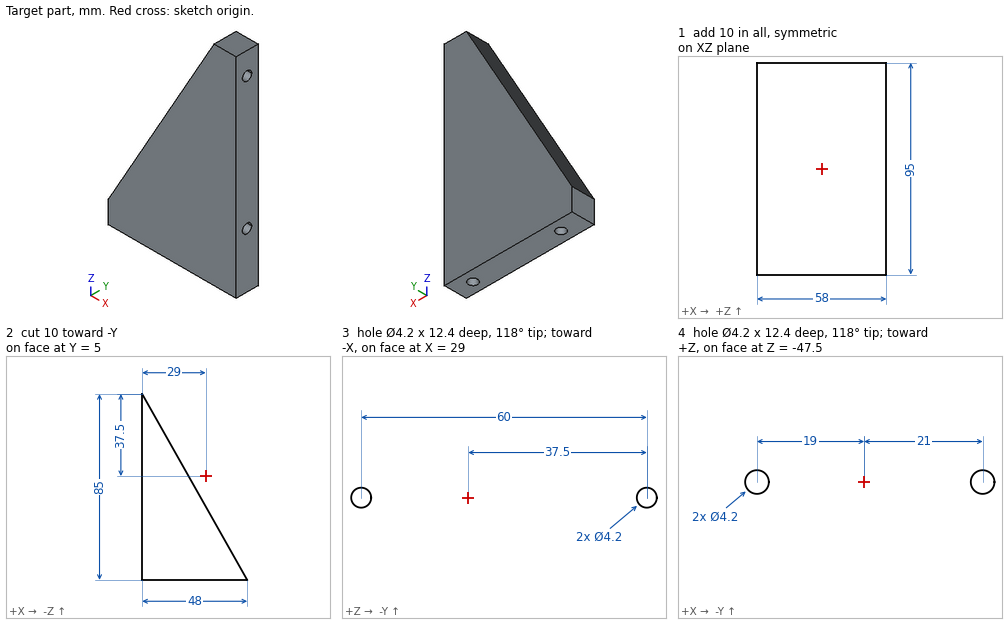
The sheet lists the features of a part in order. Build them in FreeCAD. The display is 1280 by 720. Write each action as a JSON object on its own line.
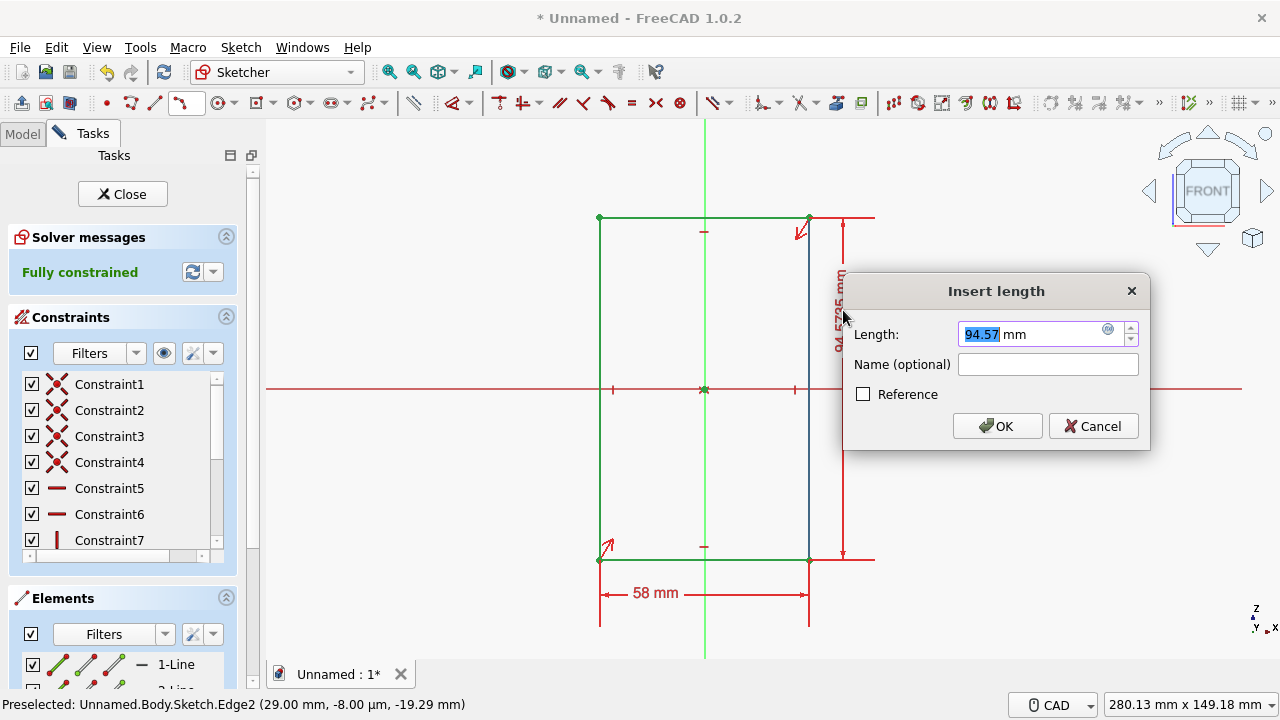
{"action": "type", "text": "95"}
{"action": "key", "text": "Return"}
{"action": "key", "text": "Escape"}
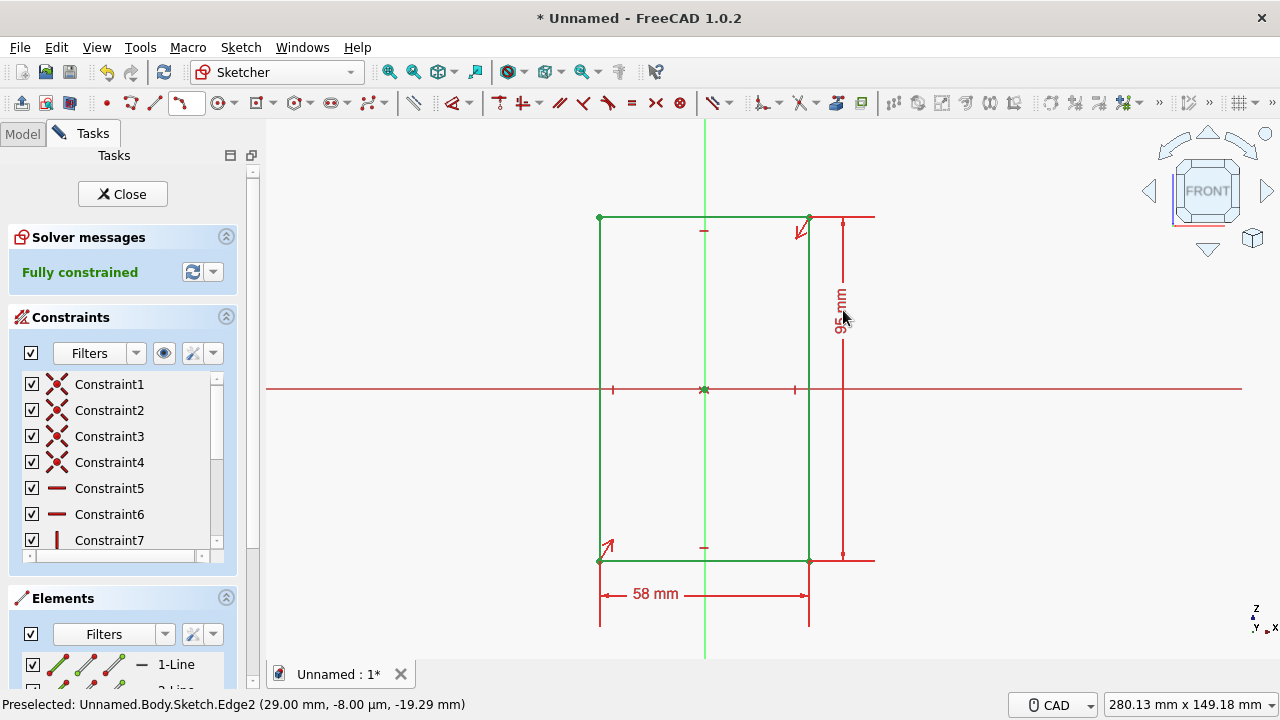
{"action": "left_click", "coordinate": [123, 194]}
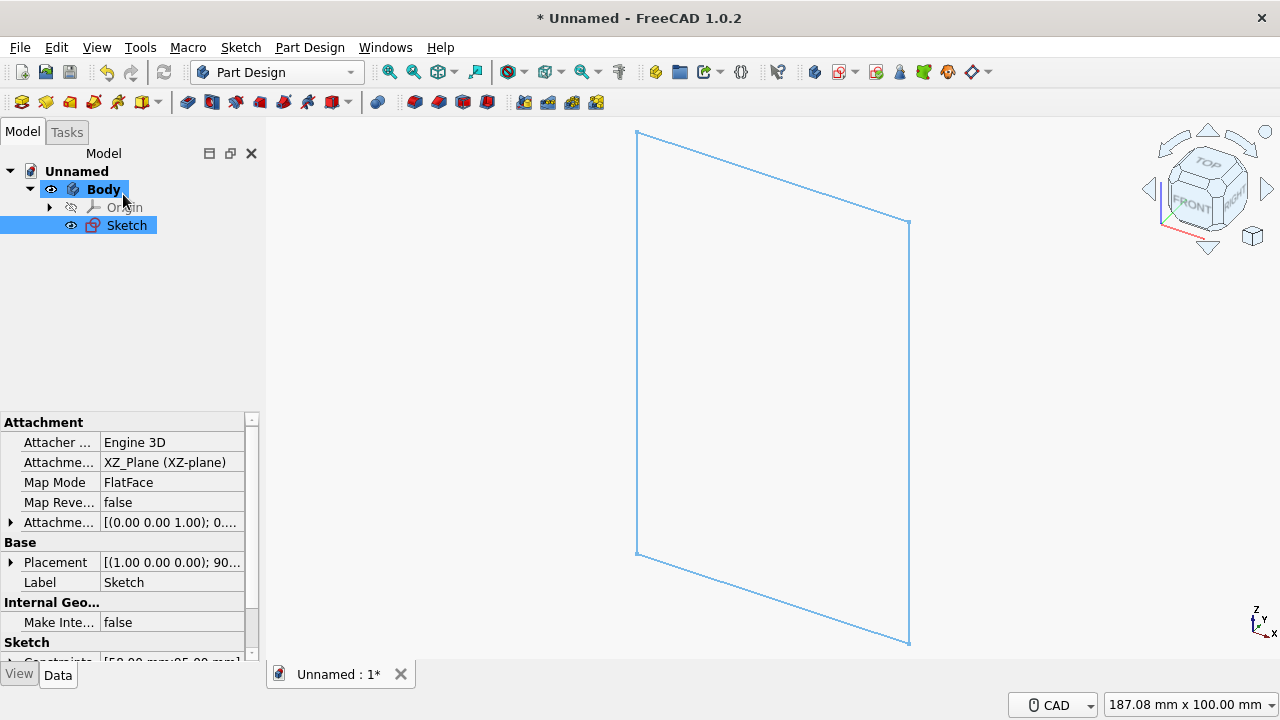
{"action": "left_click", "coordinate": [22, 102]}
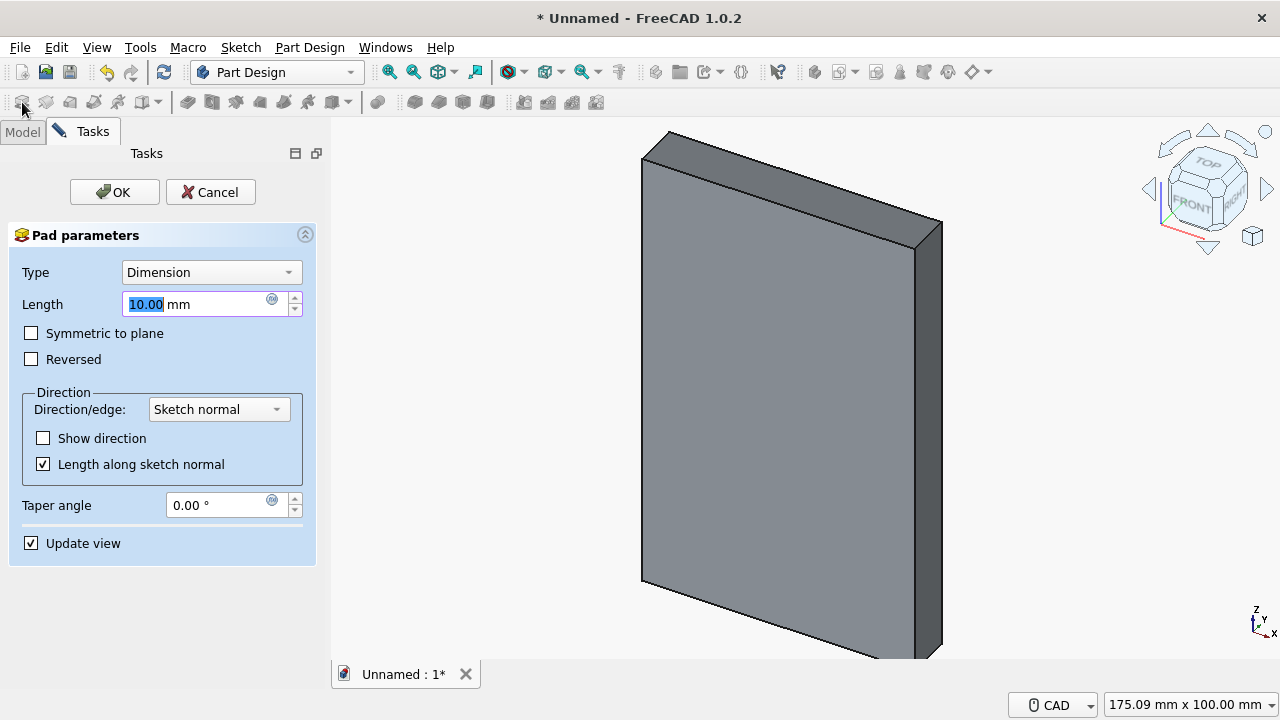
{"action": "type", "text": "10"}
{"action": "key", "text": "Tab"}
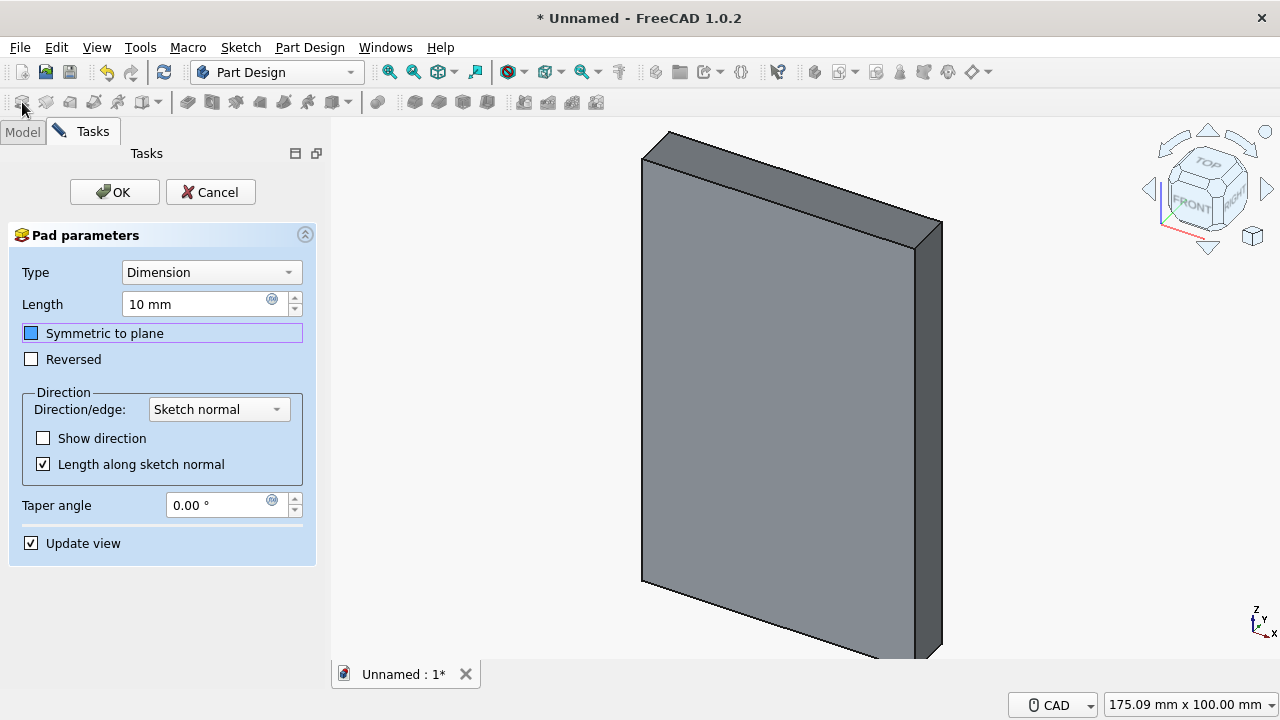
{"action": "left_click", "coordinate": [30, 333]}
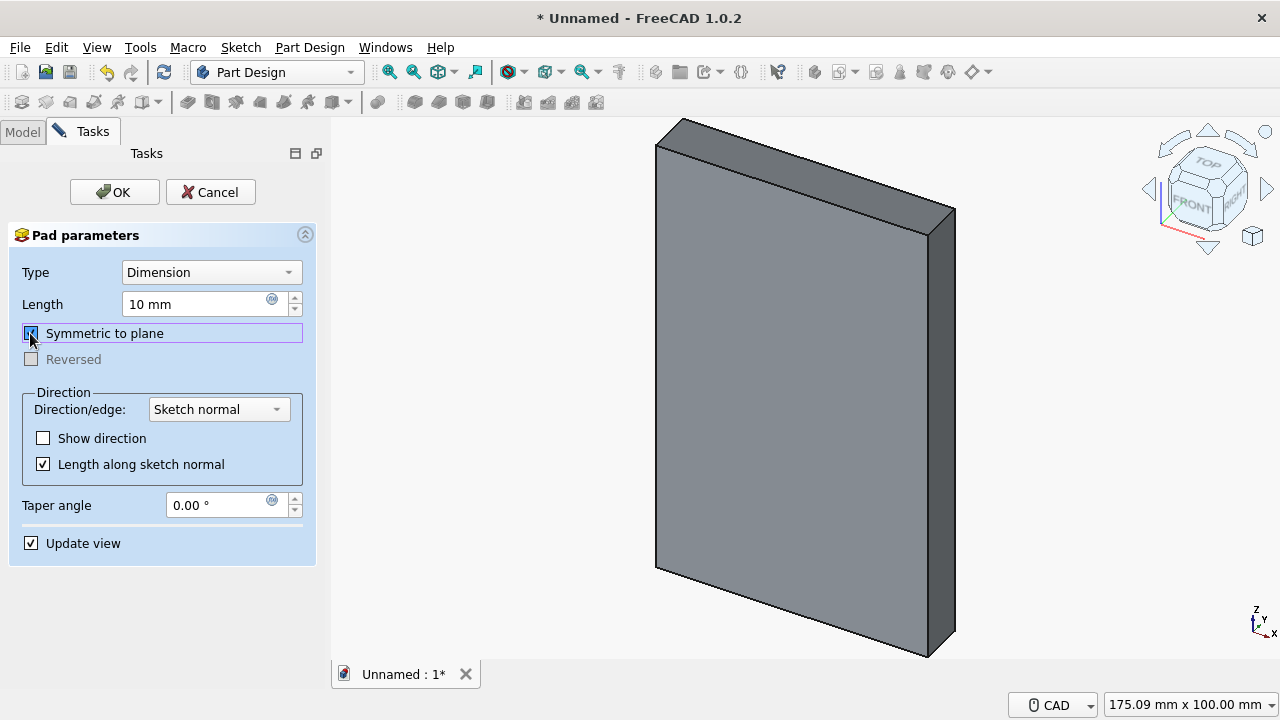
{"action": "left_click", "coordinate": [115, 192]}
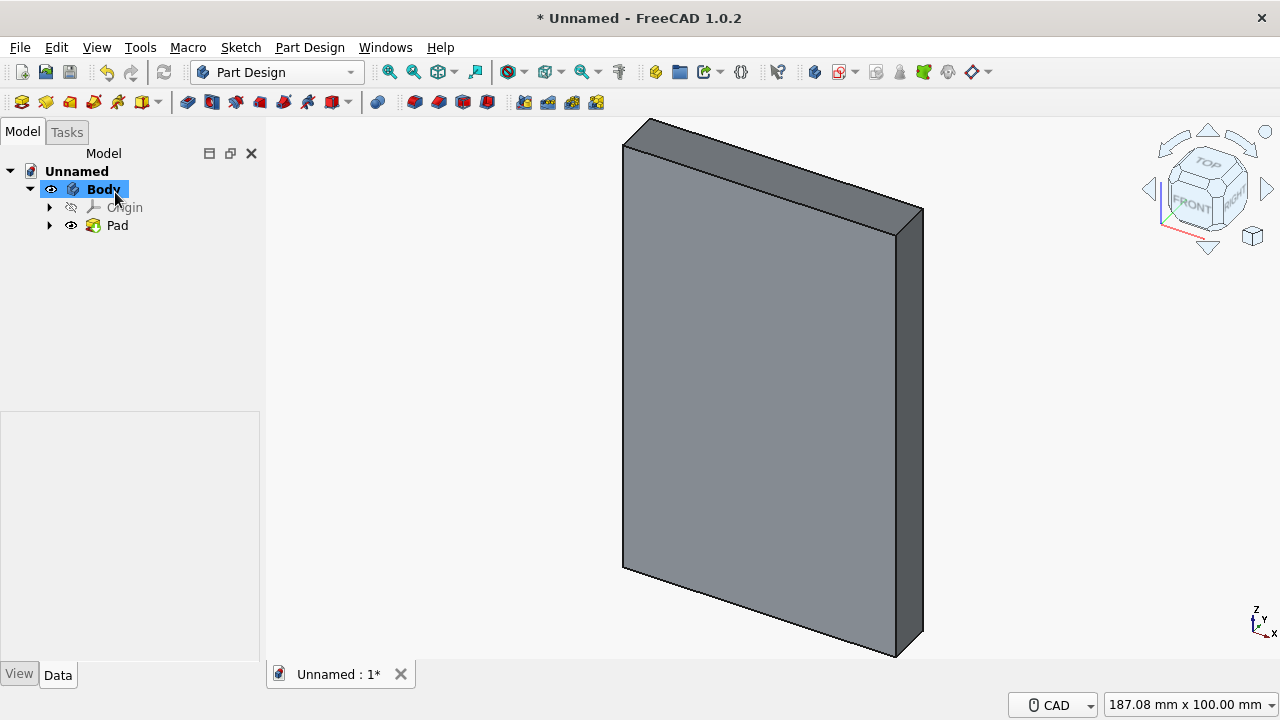
{"action": "key", "text": "4"}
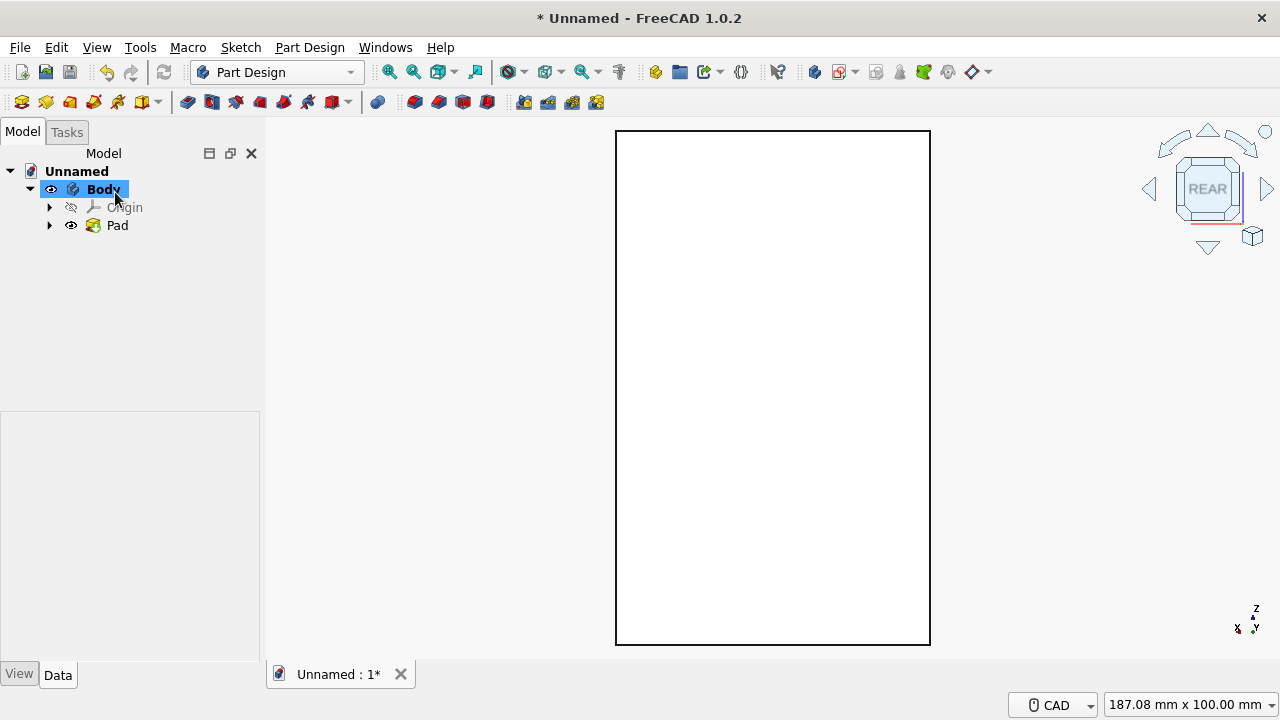
{"action": "left_click", "coordinate": [773, 313]}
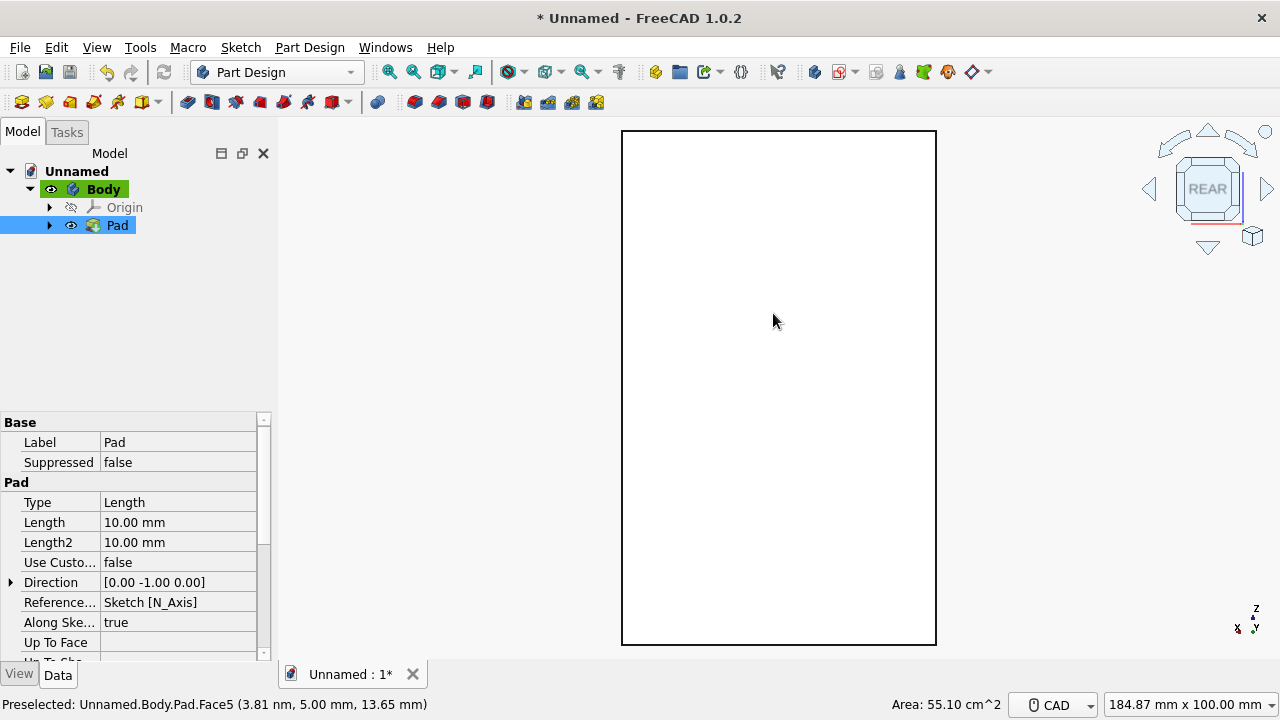
{"action": "left_click", "coordinate": [840, 72]}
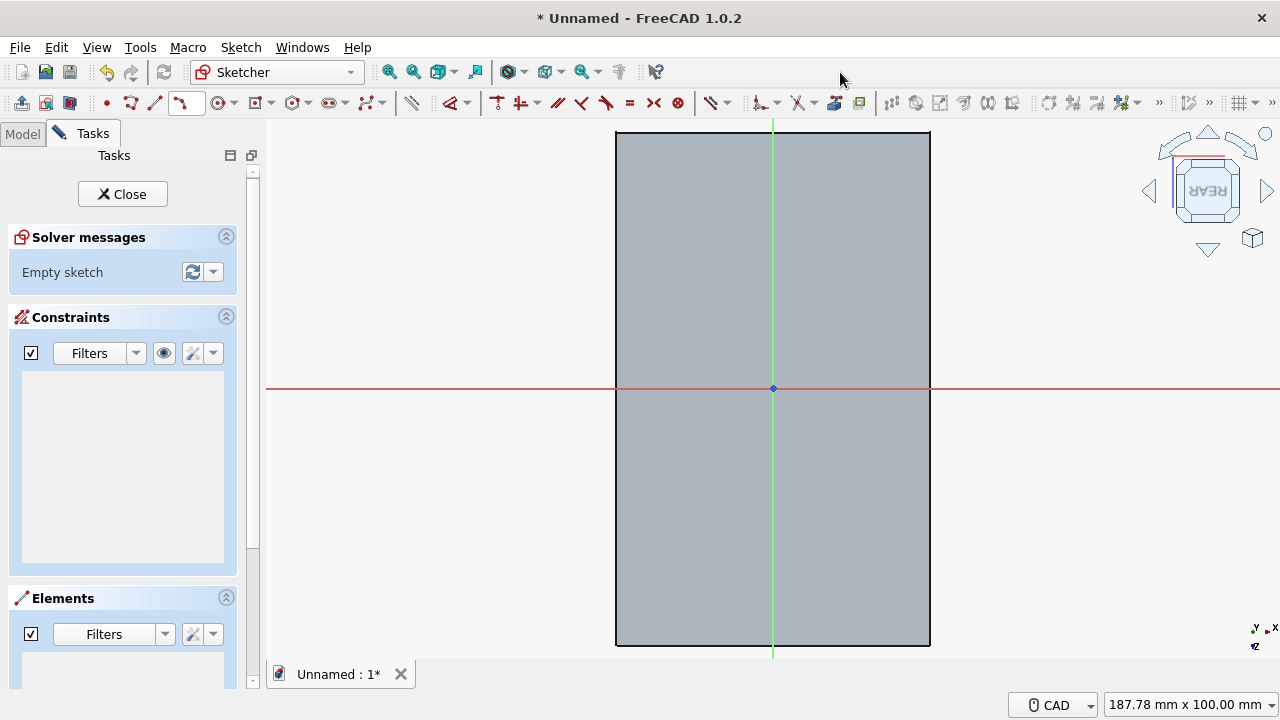
{"action": "scroll", "coordinate": [517, 267], "scroll_direction": "down", "scroll_amount": 1}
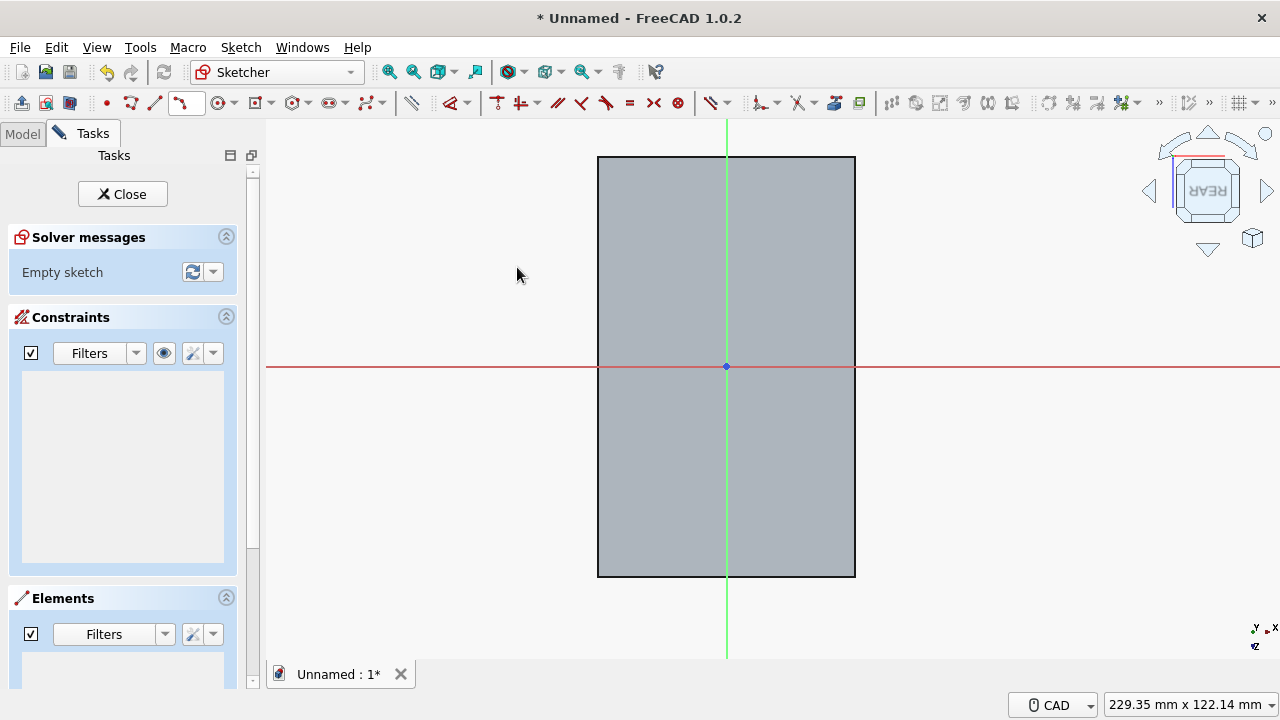
{"action": "left_click", "coordinate": [132, 104]}